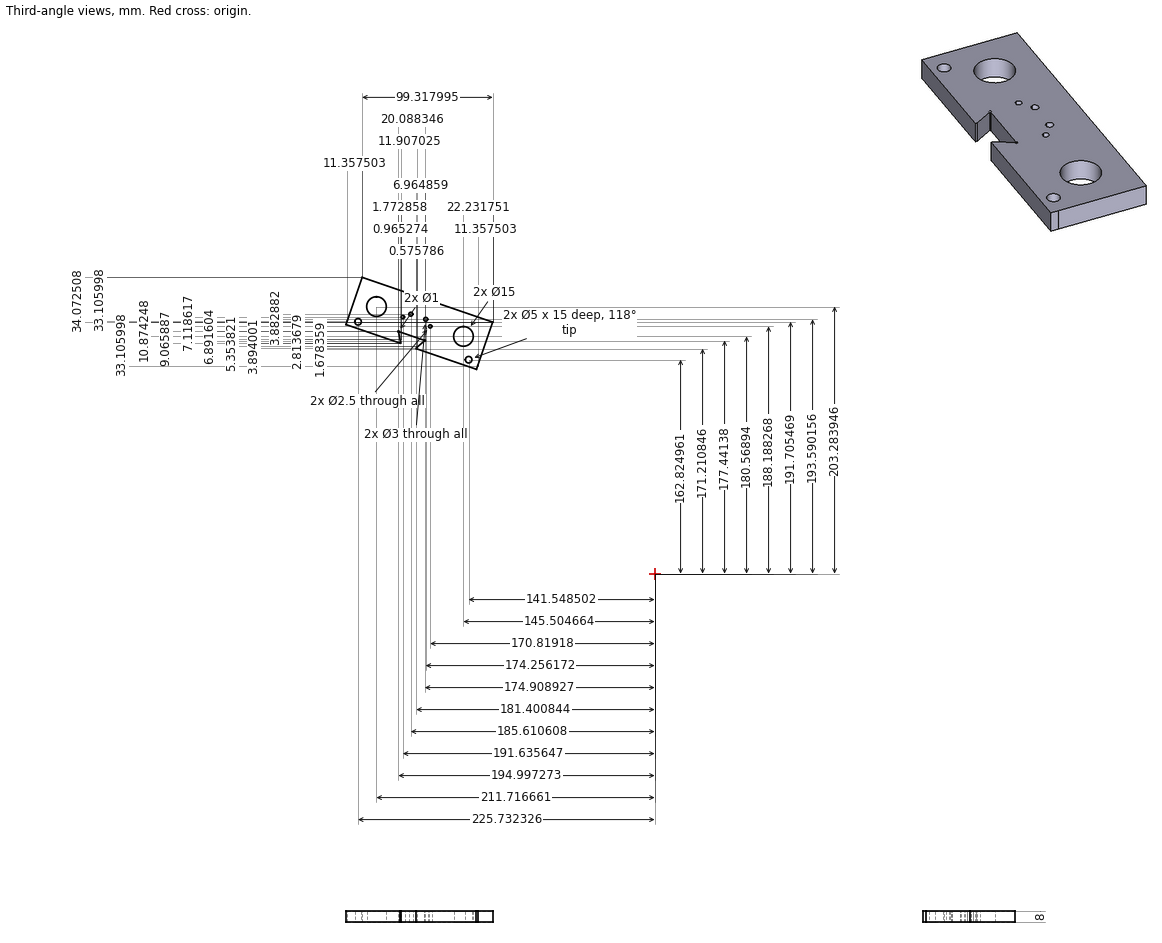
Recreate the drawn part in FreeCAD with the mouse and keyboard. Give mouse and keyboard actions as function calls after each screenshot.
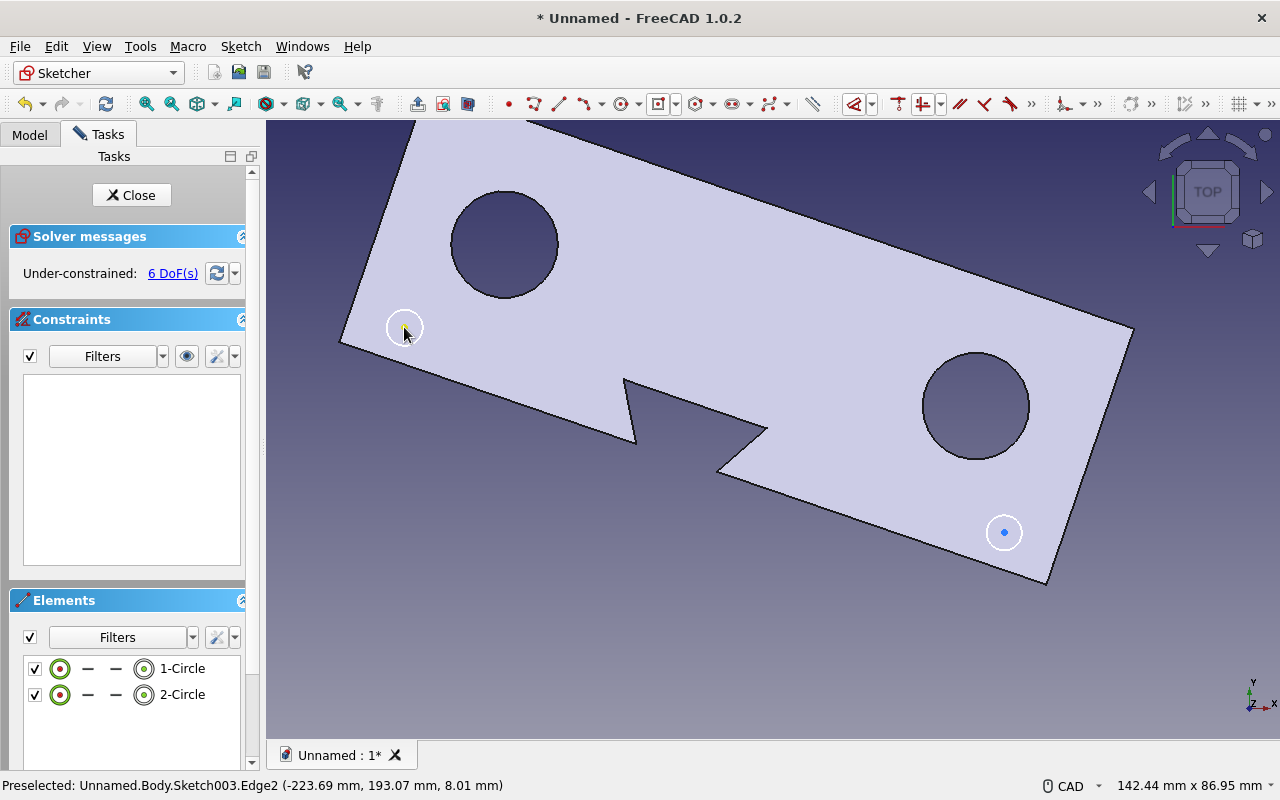
click(1017, 520)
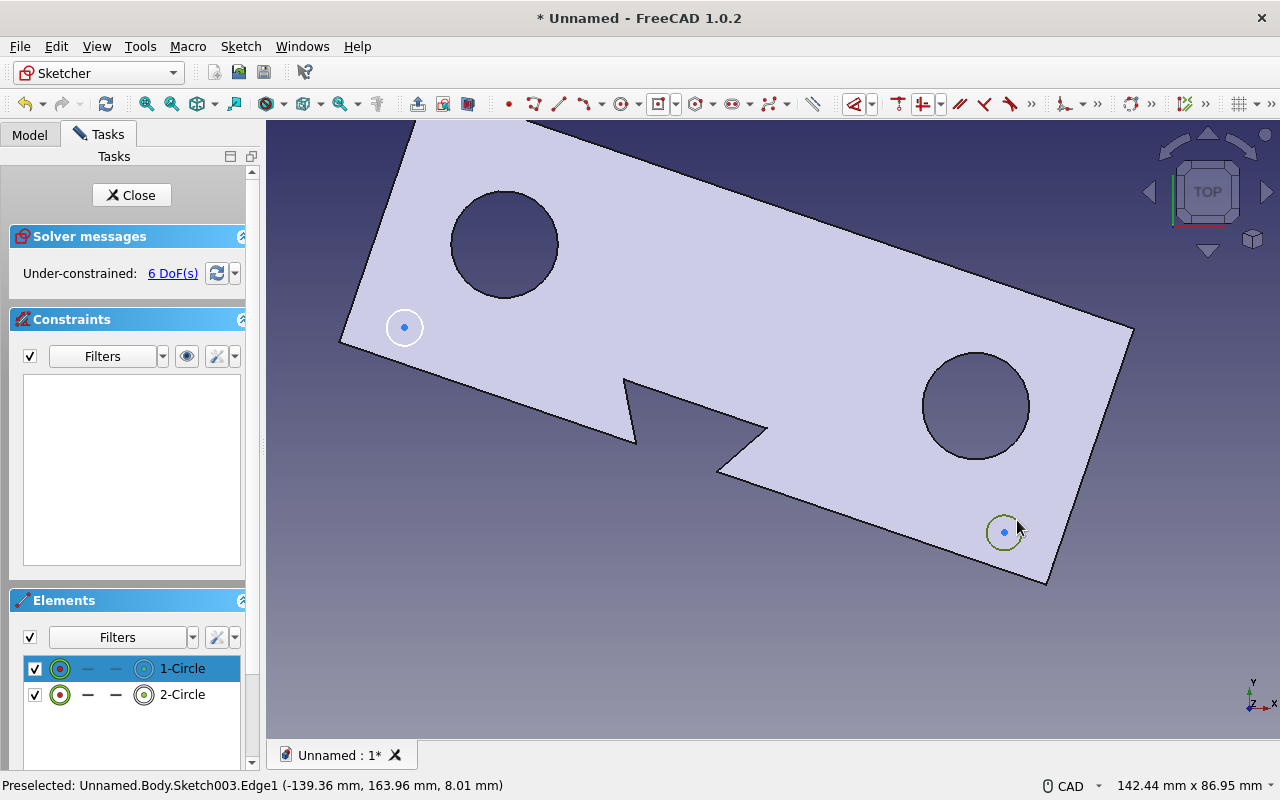
click(417, 315)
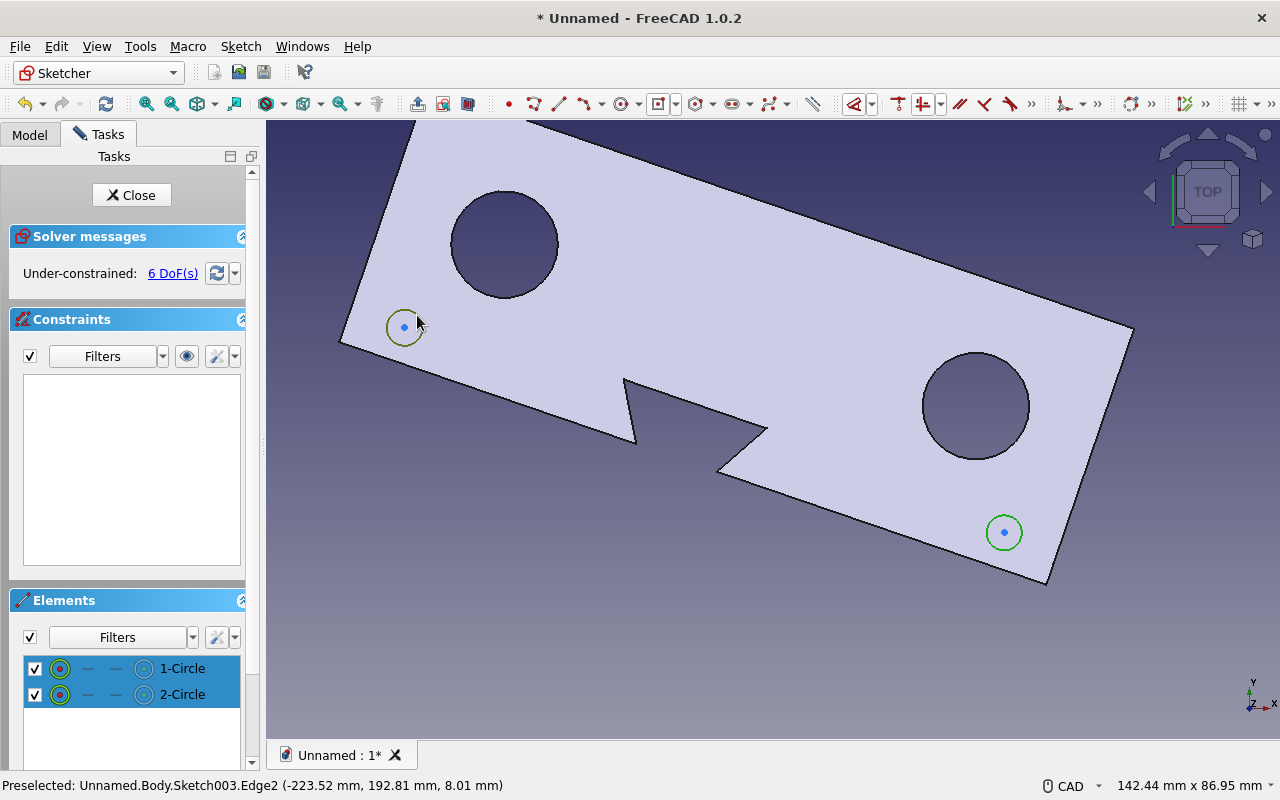
key(e)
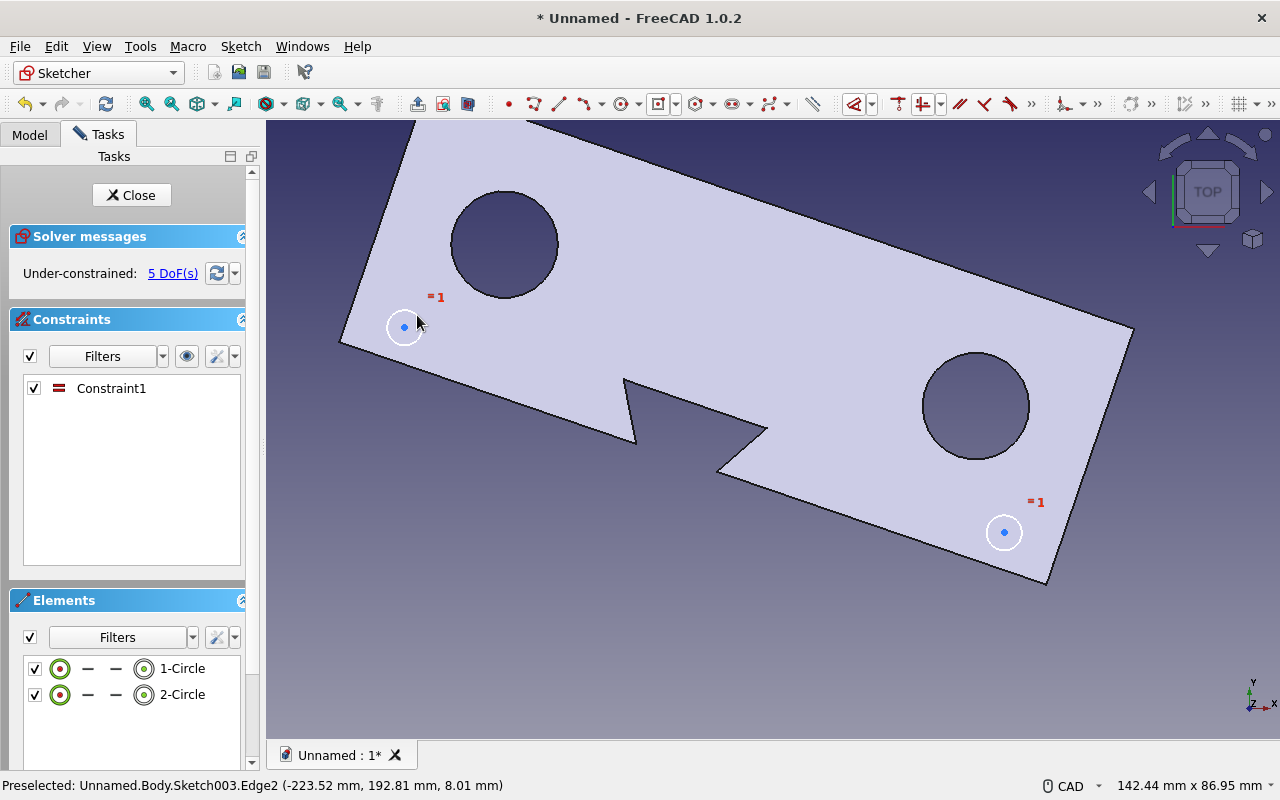
click(1017, 520)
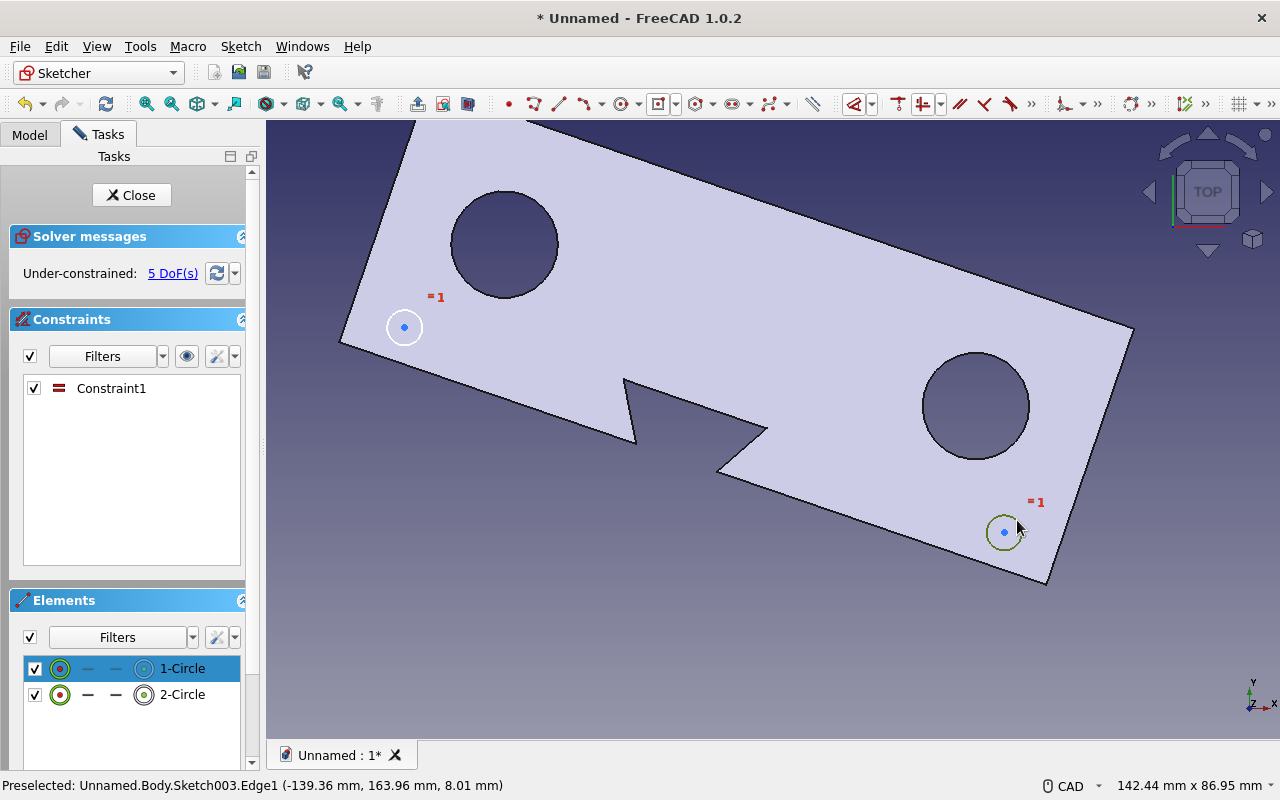
key(k)
key(o)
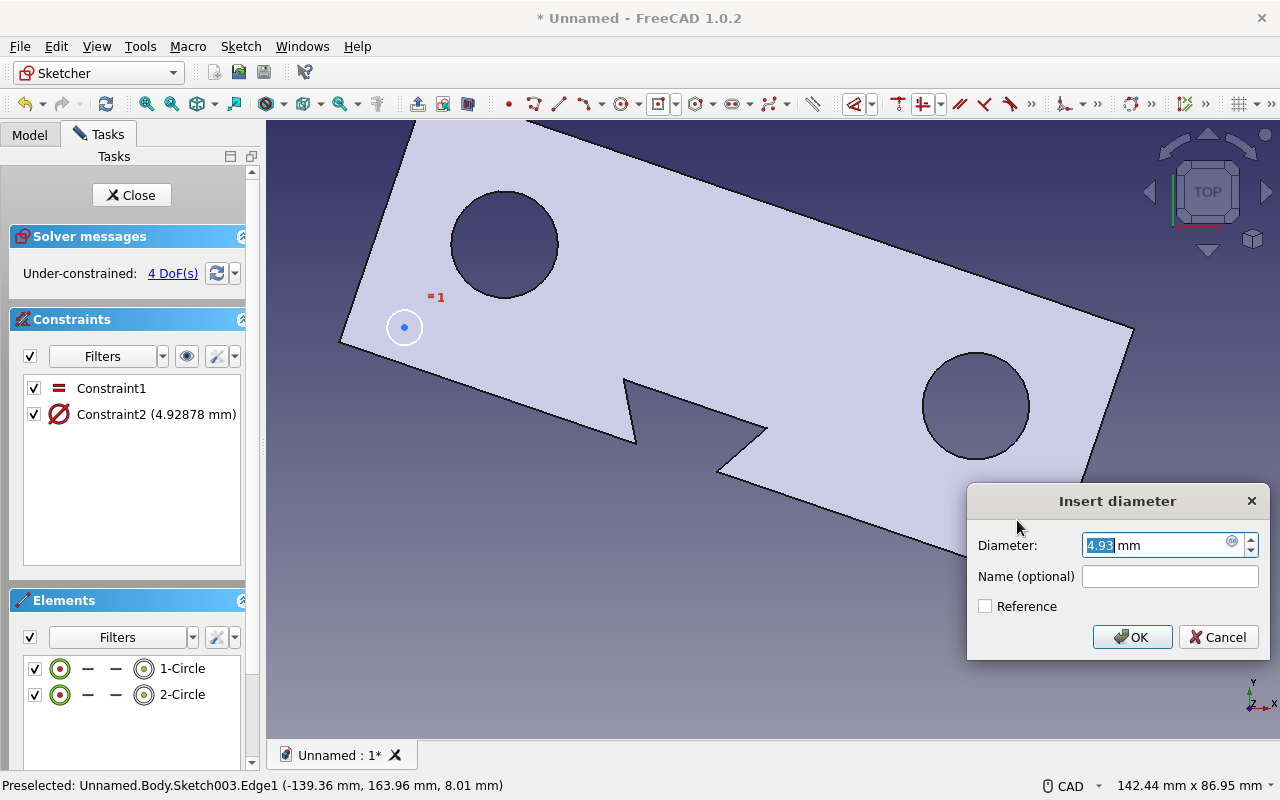
text(5)
key(Return)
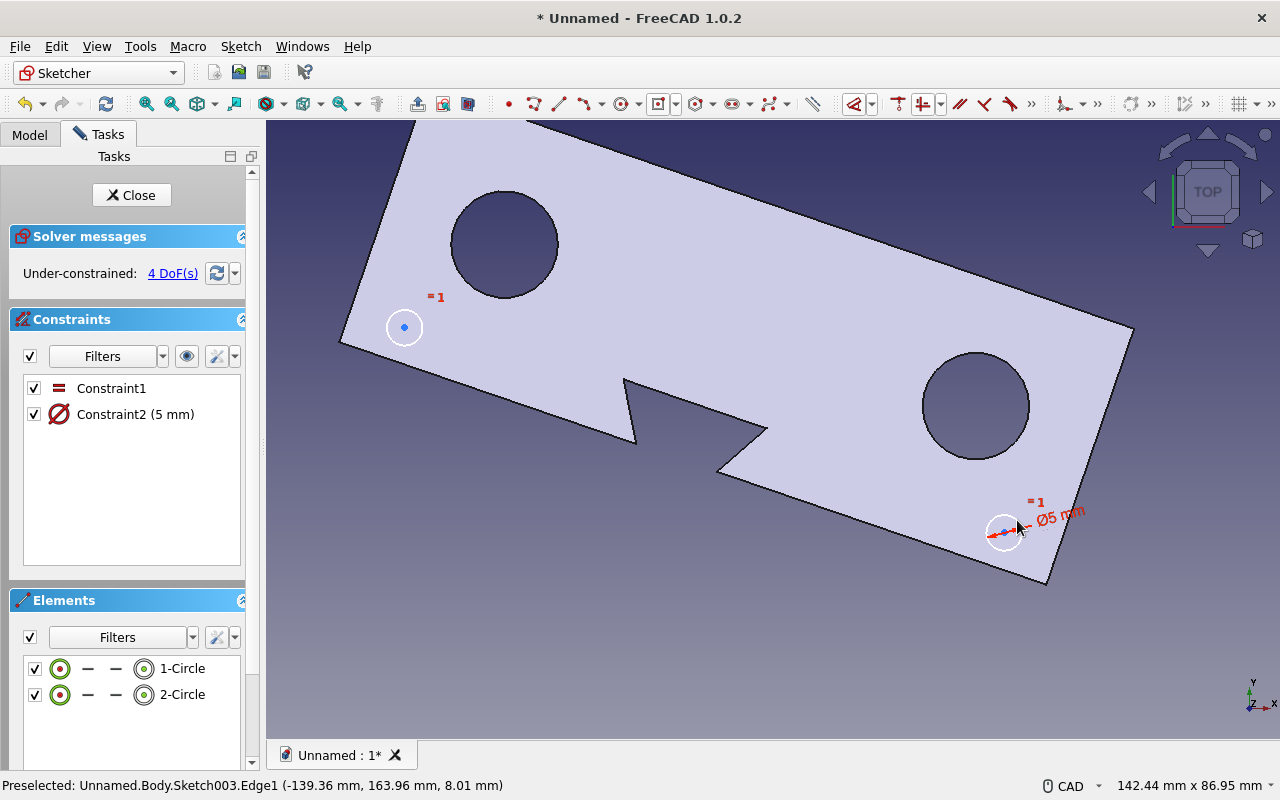
click(1004, 533)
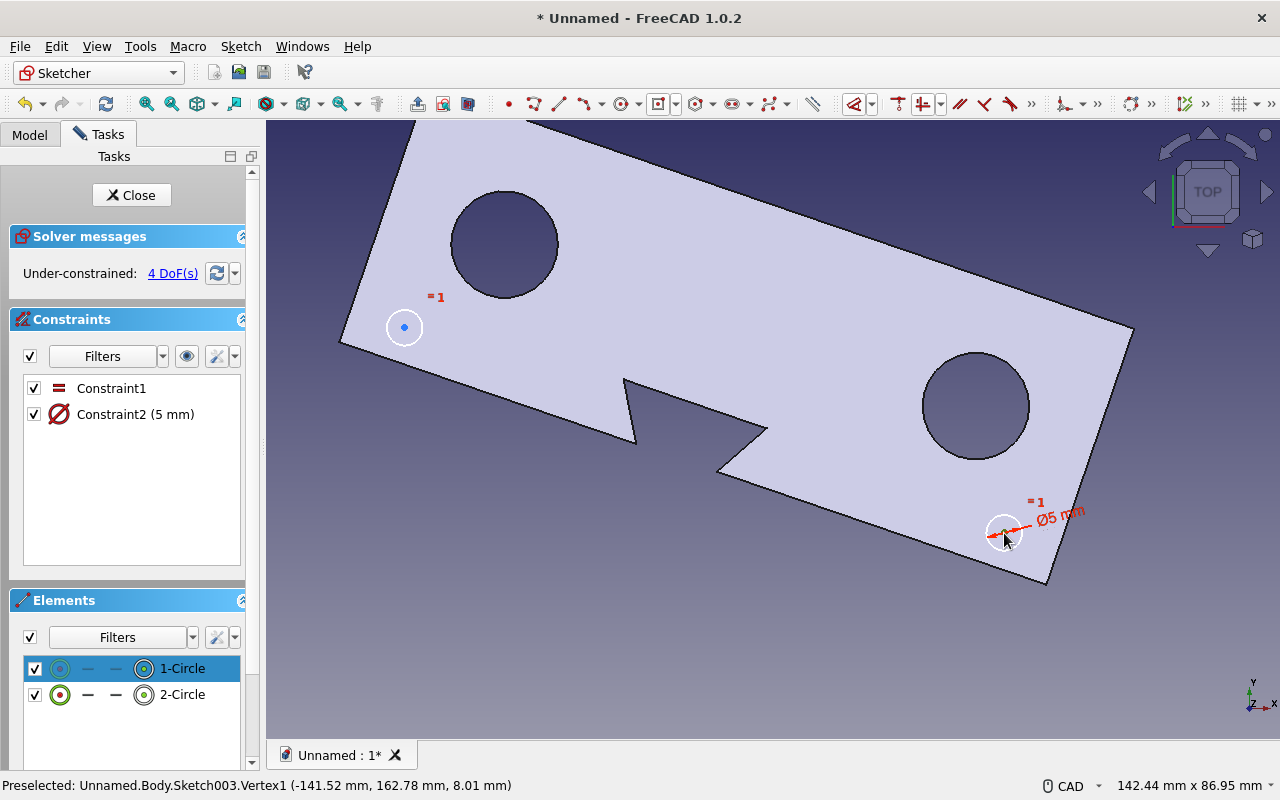
key(l)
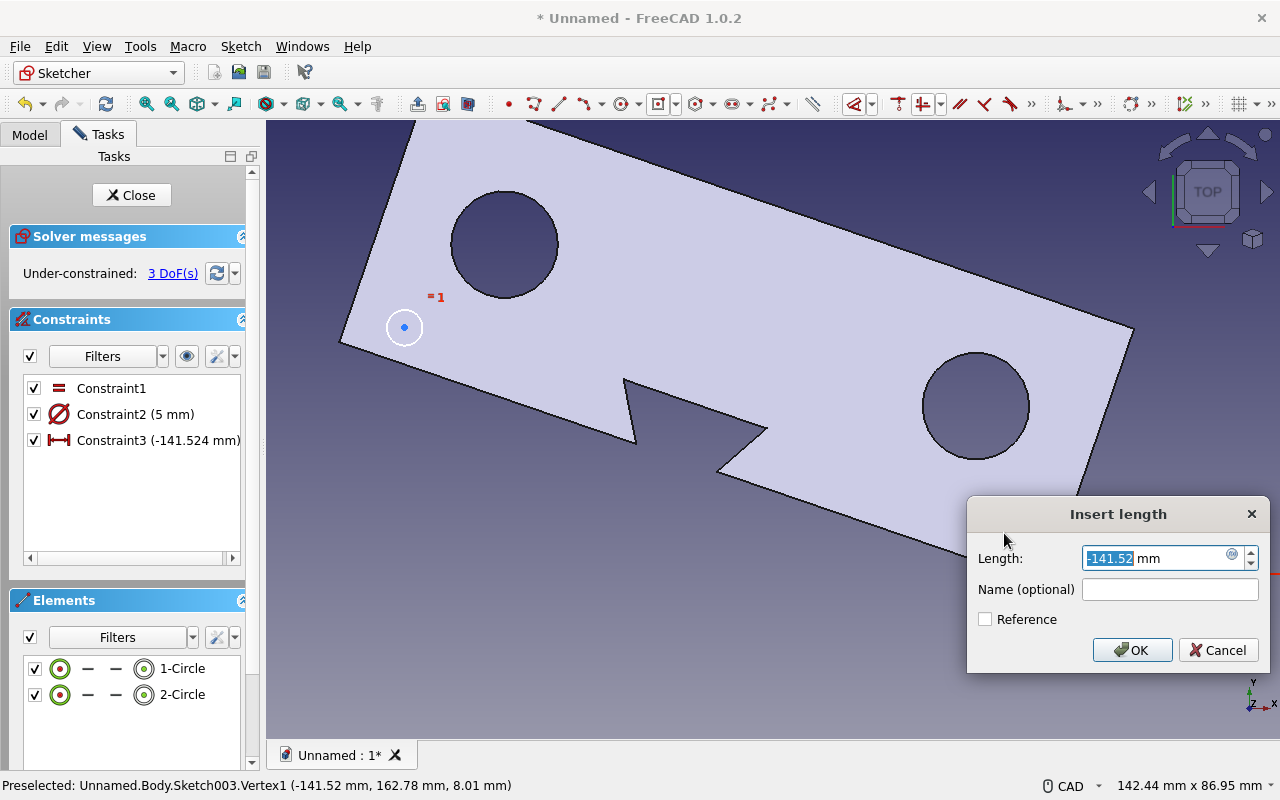
text(-141.548502)
key(Return)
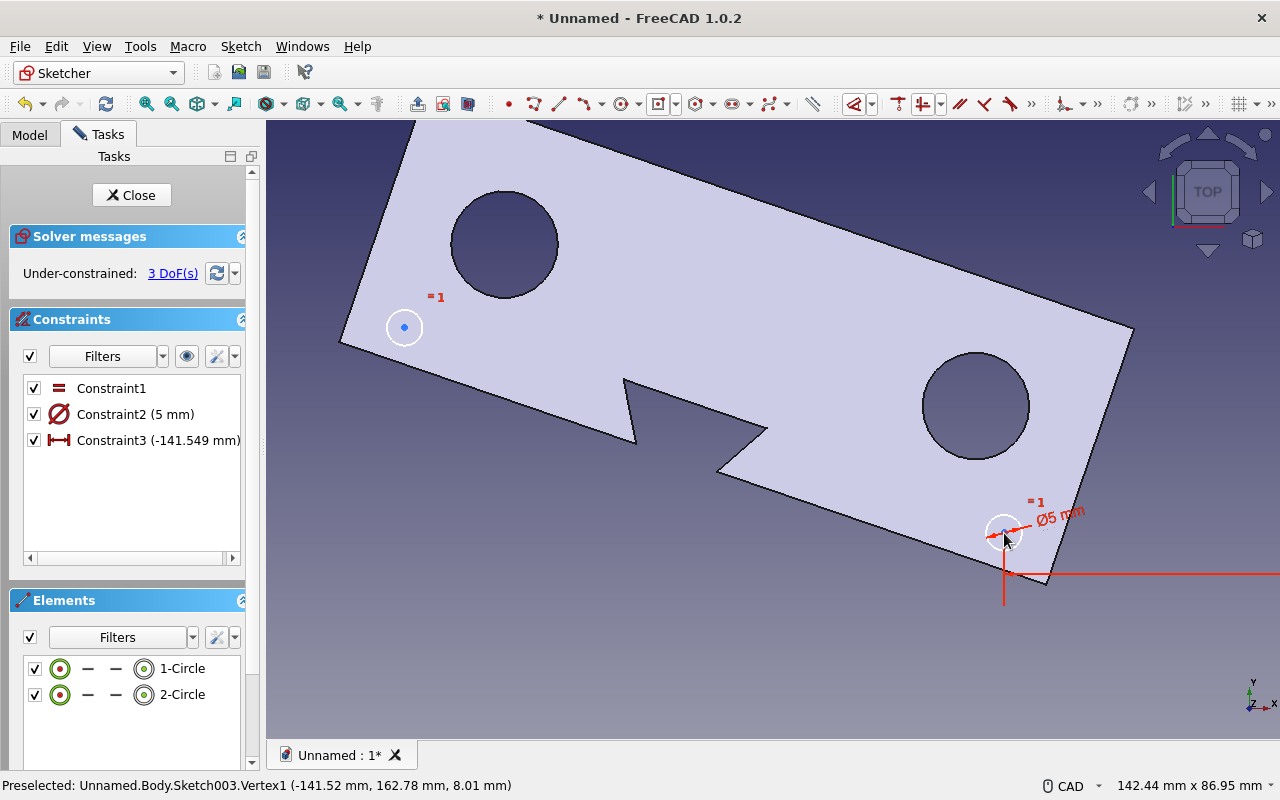
click(1004, 533)